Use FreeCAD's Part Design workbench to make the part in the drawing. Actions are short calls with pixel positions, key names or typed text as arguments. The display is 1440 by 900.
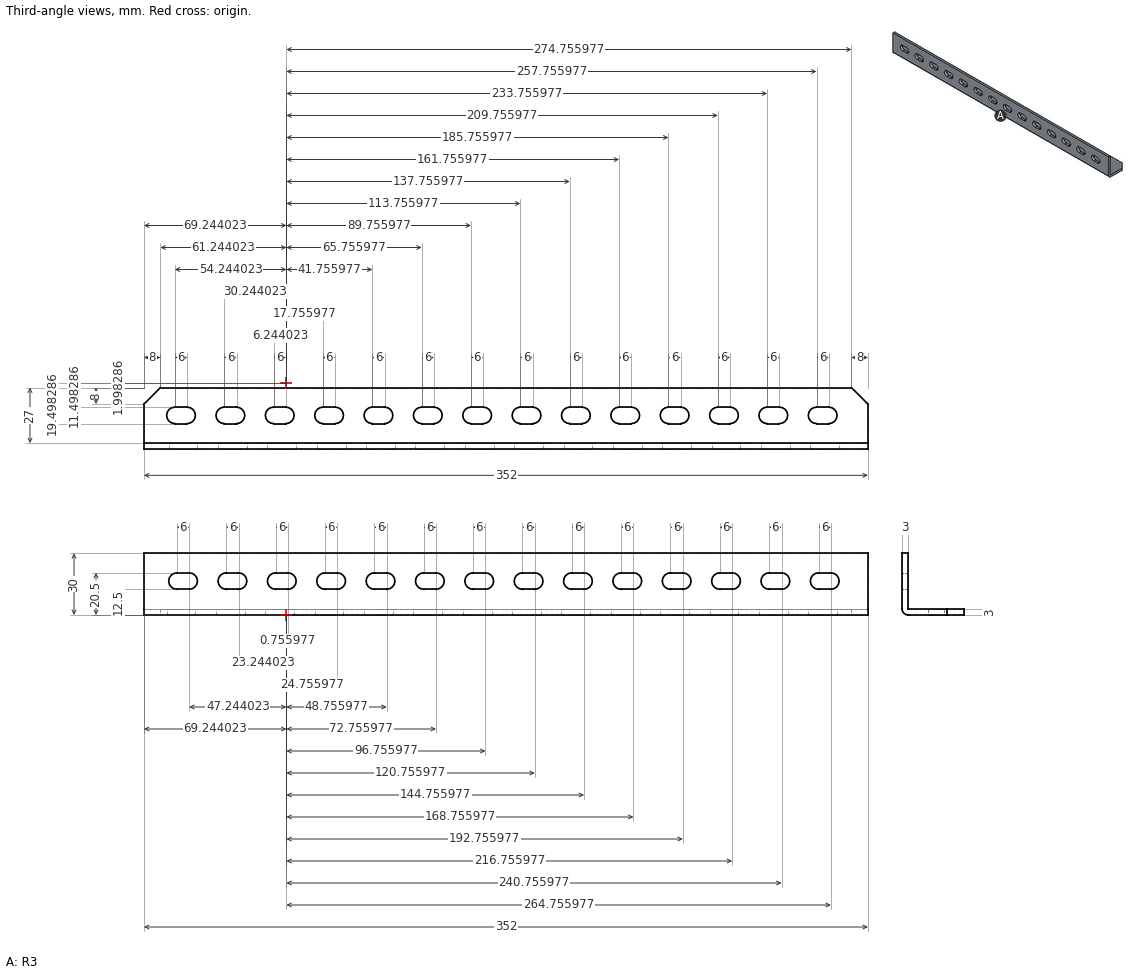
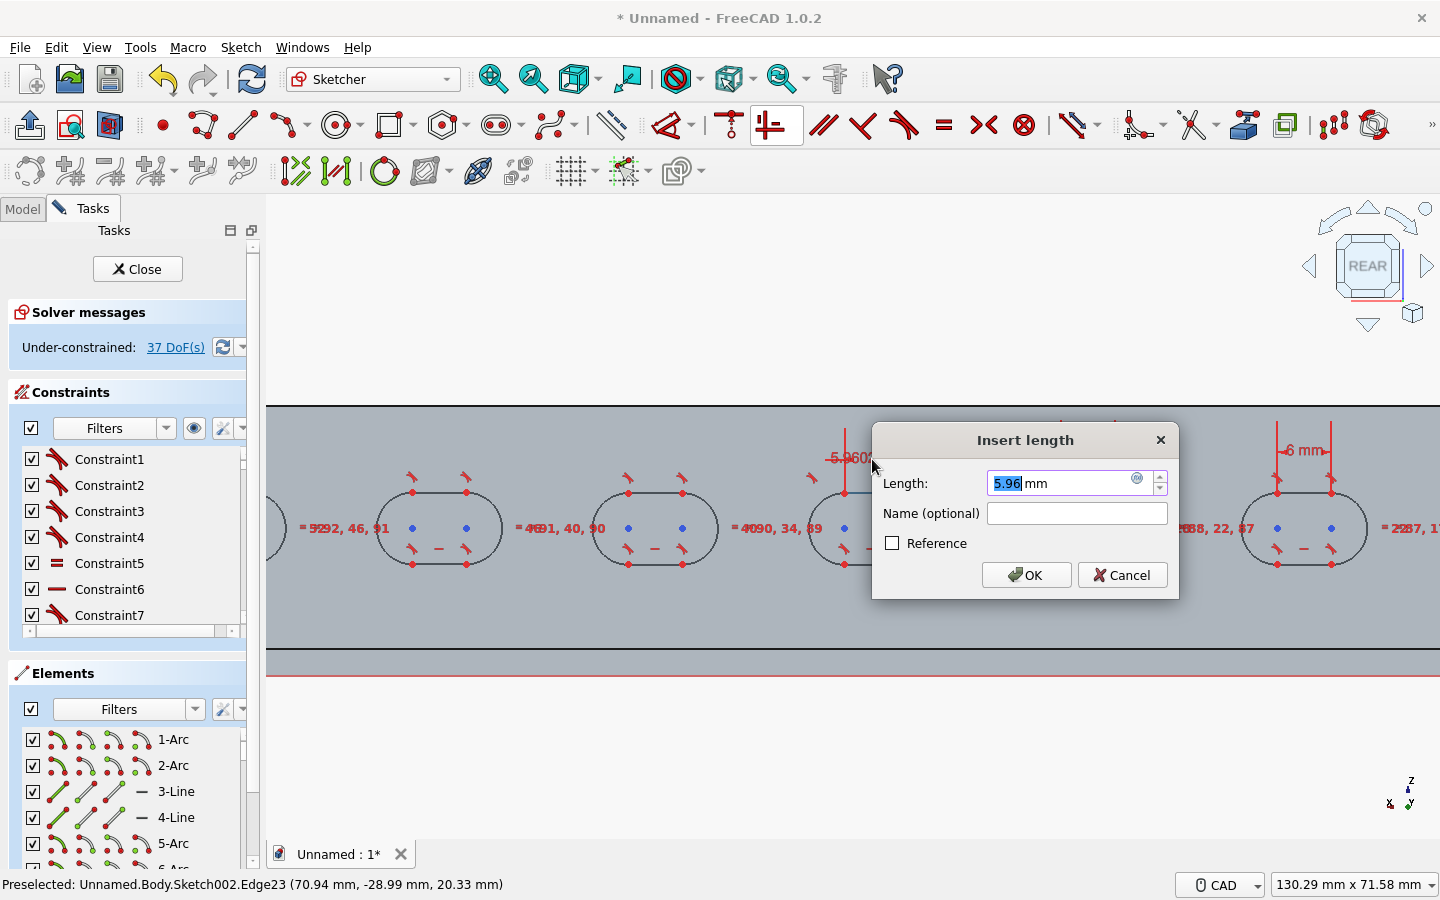
text(6)
key(Return)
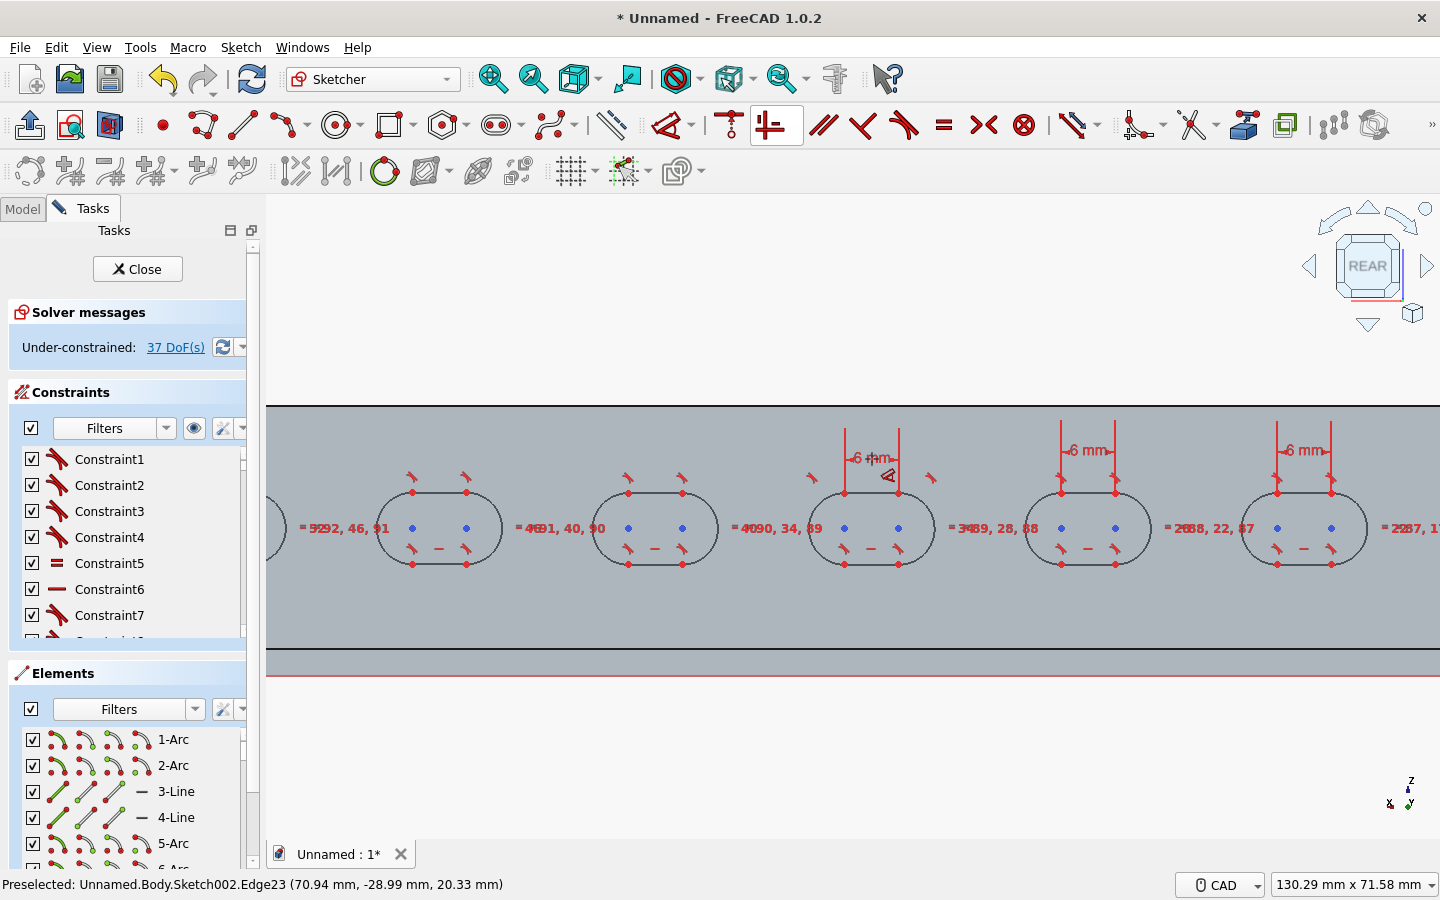
click(645, 493)
click(655, 459)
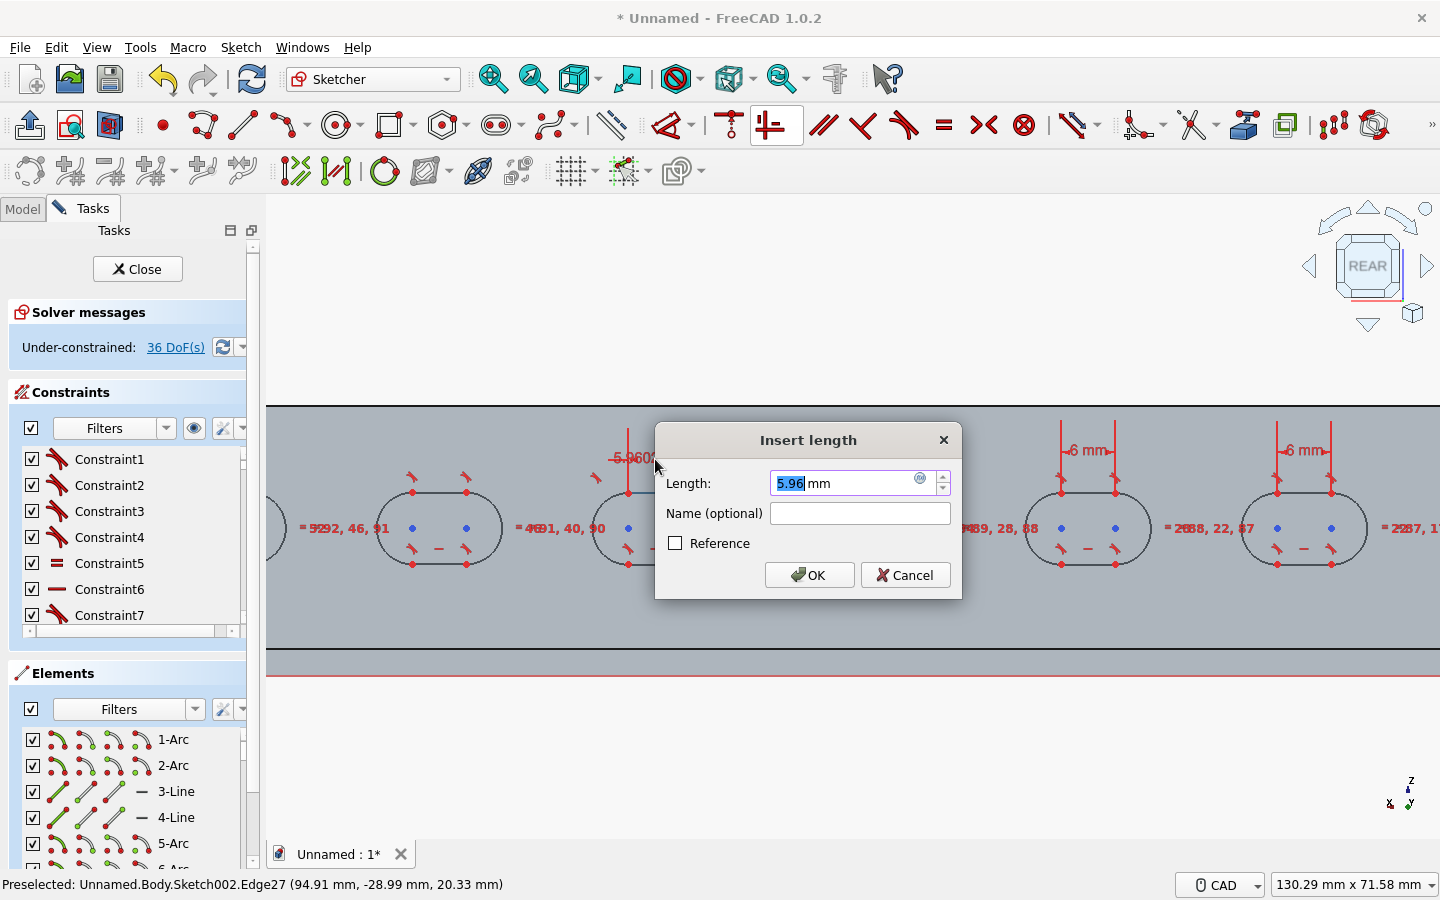
text(6)
key(Return)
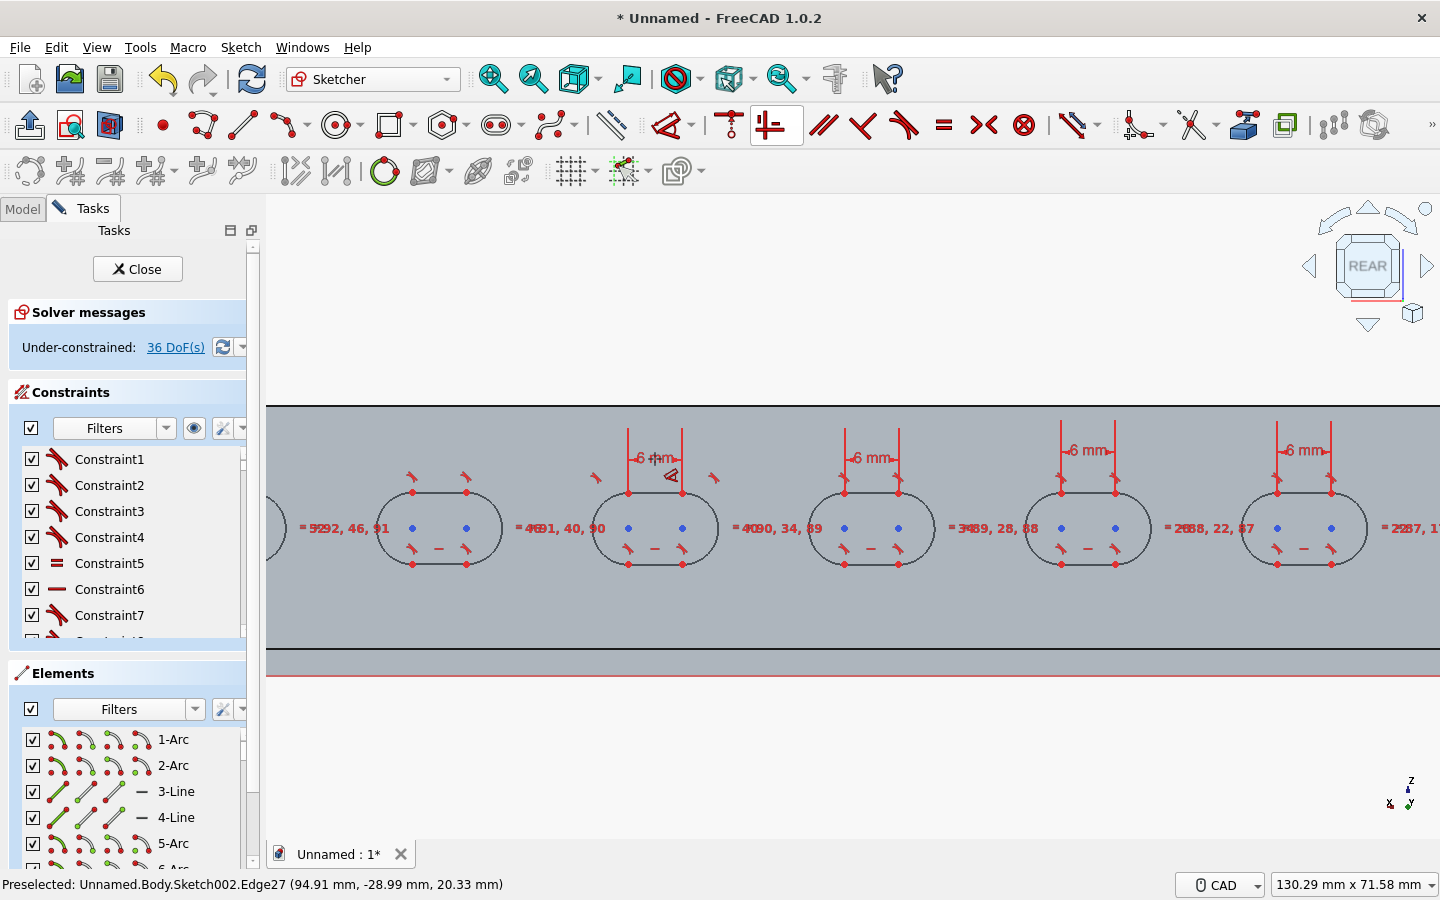
click(429, 493)
click(439, 459)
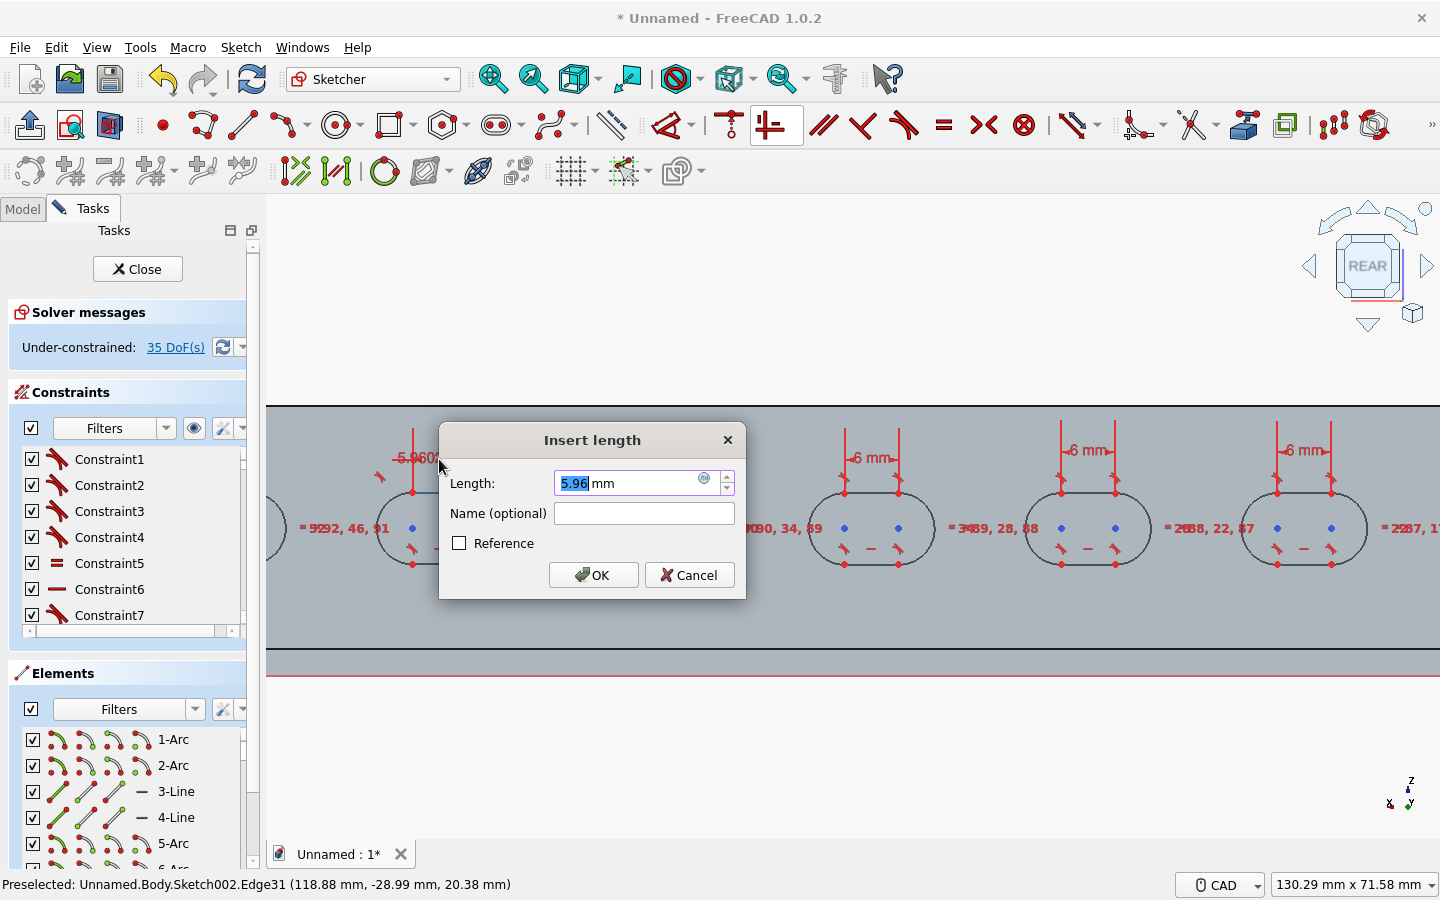
text(6)
key(Return)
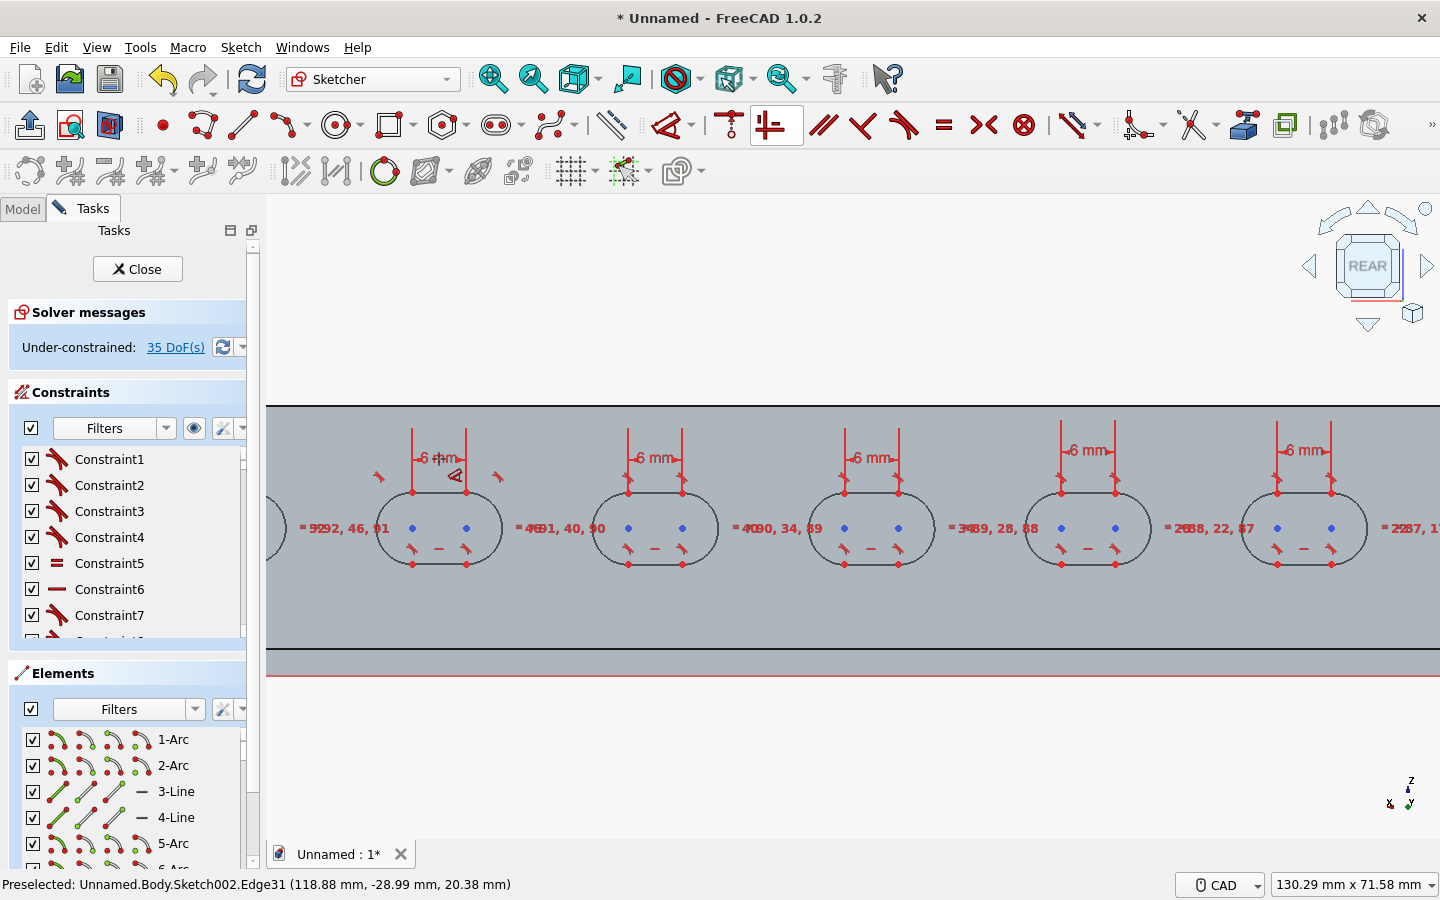
scroll(862, 494, down, 7)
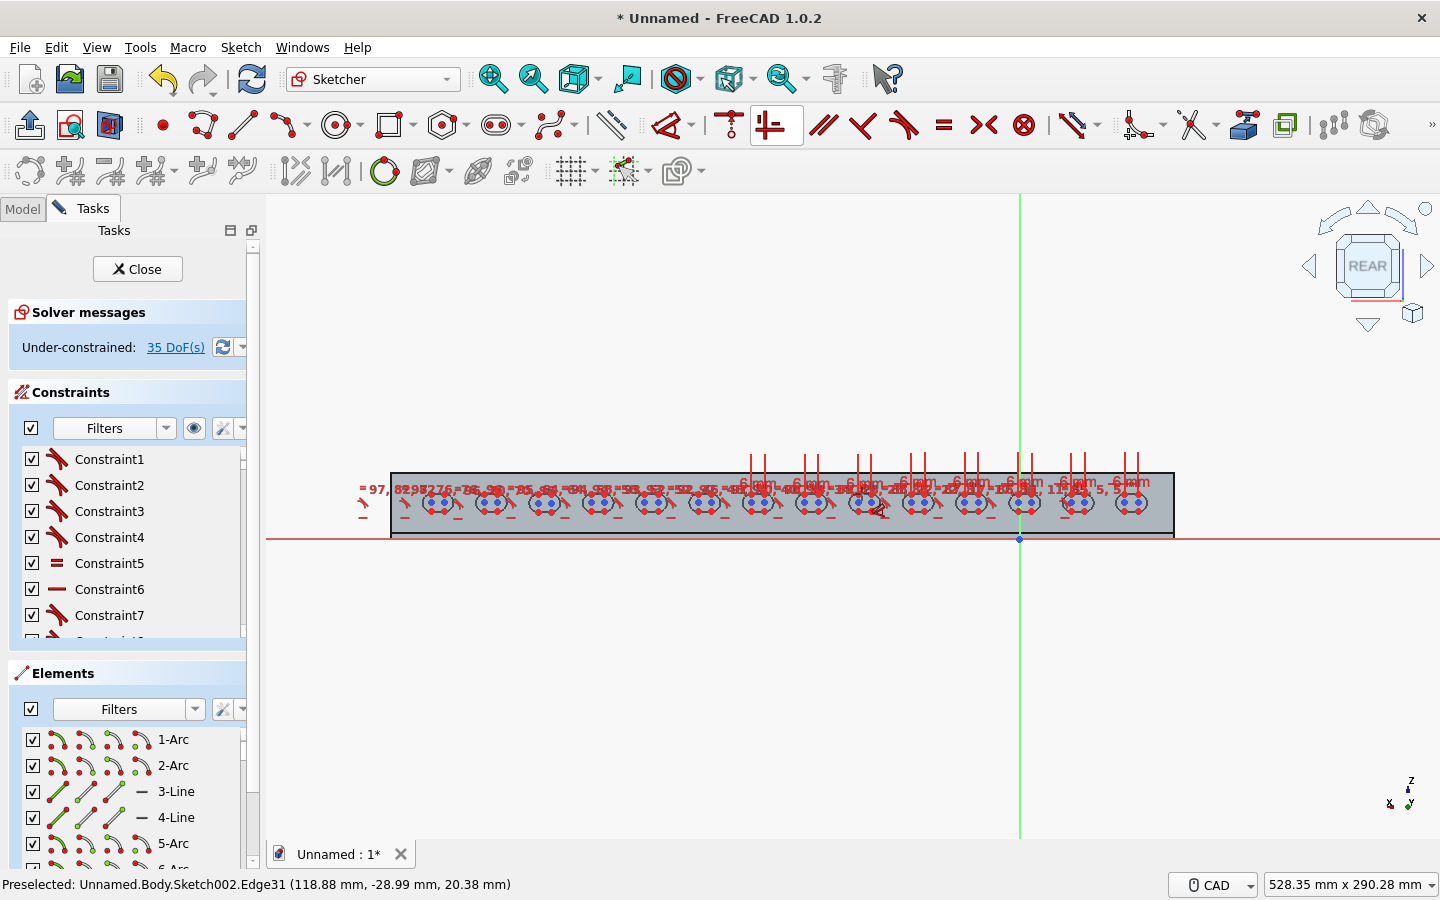
scroll(702, 494, up, 7)